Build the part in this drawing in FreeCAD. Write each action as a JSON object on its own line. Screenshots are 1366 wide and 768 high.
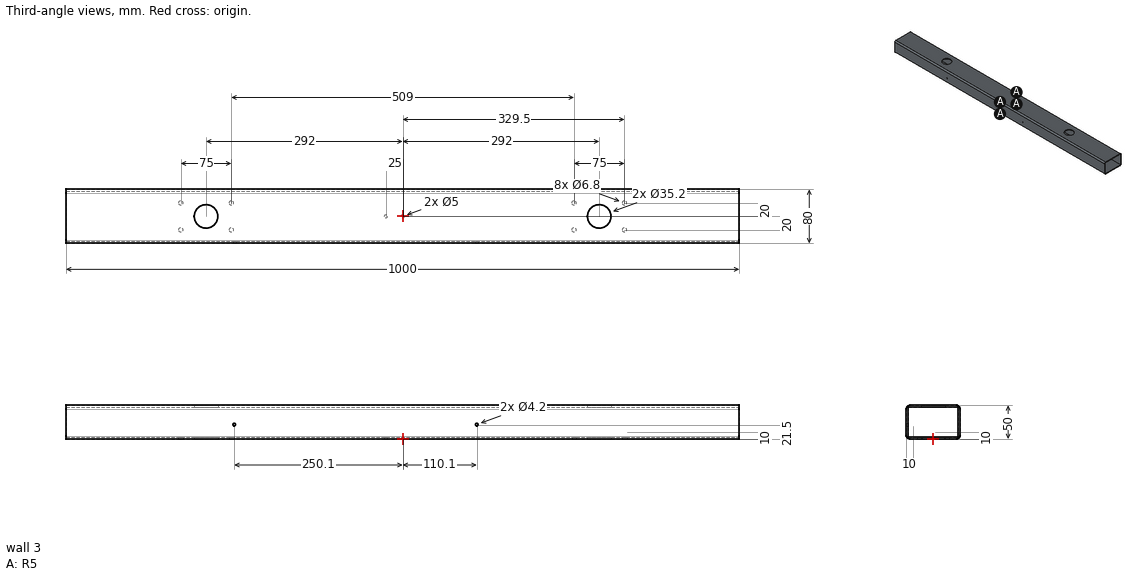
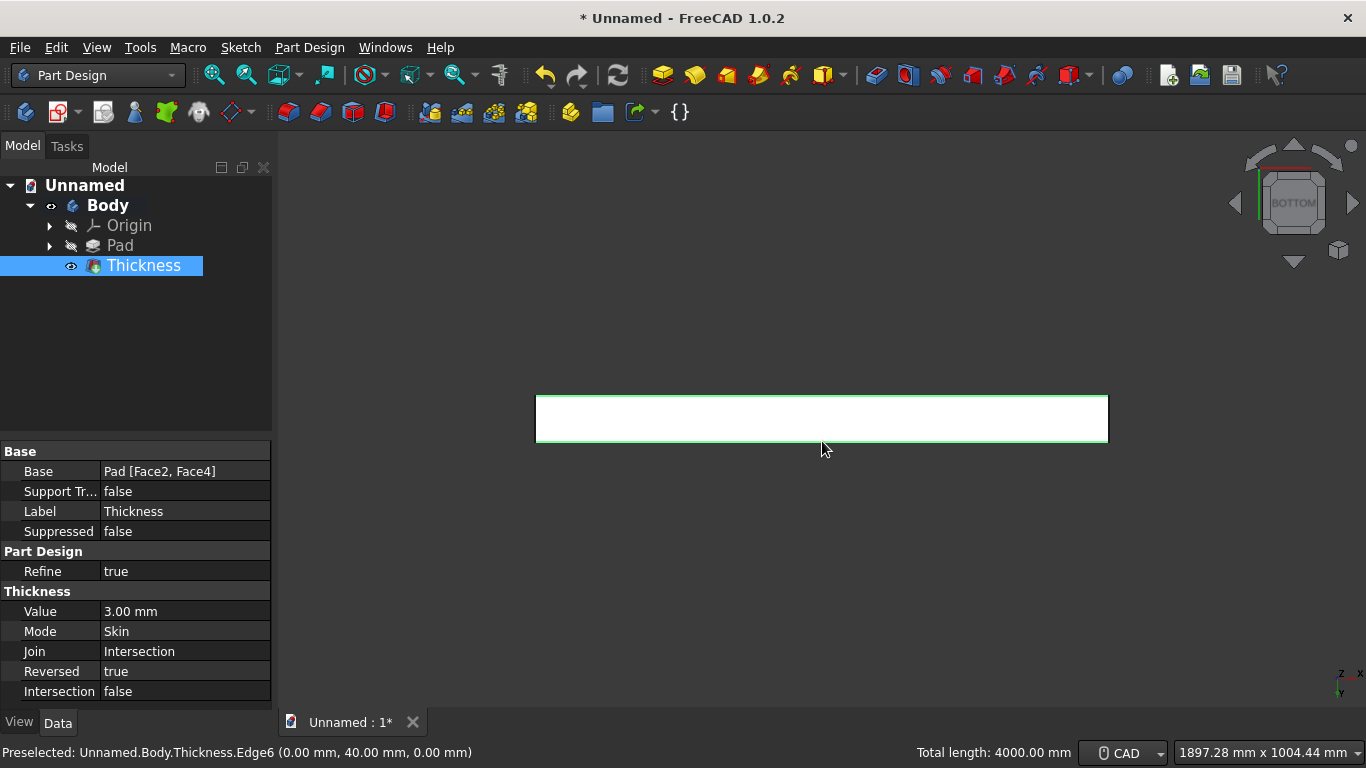
{"action": "left_click", "coordinate": [290, 112]}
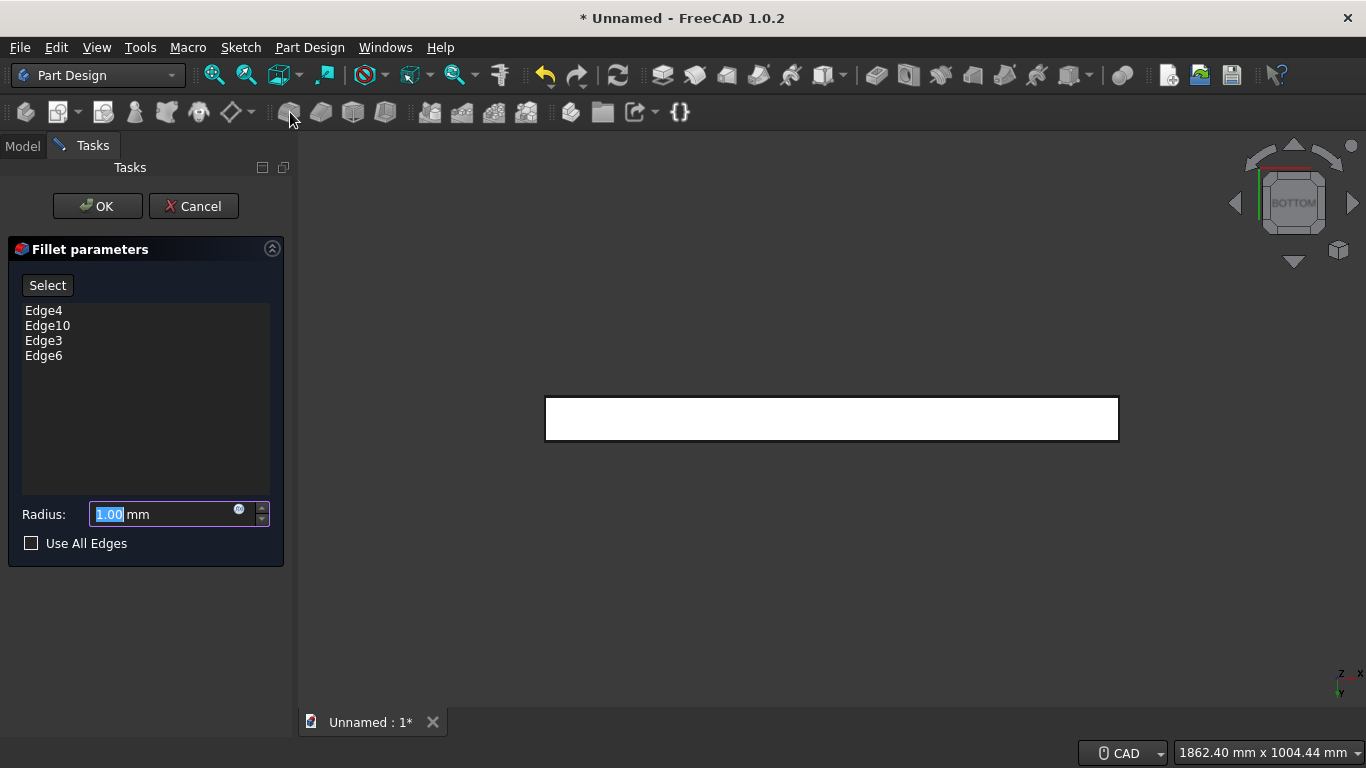
{"action": "type", "text": "5"}
{"action": "key", "text": "Tab"}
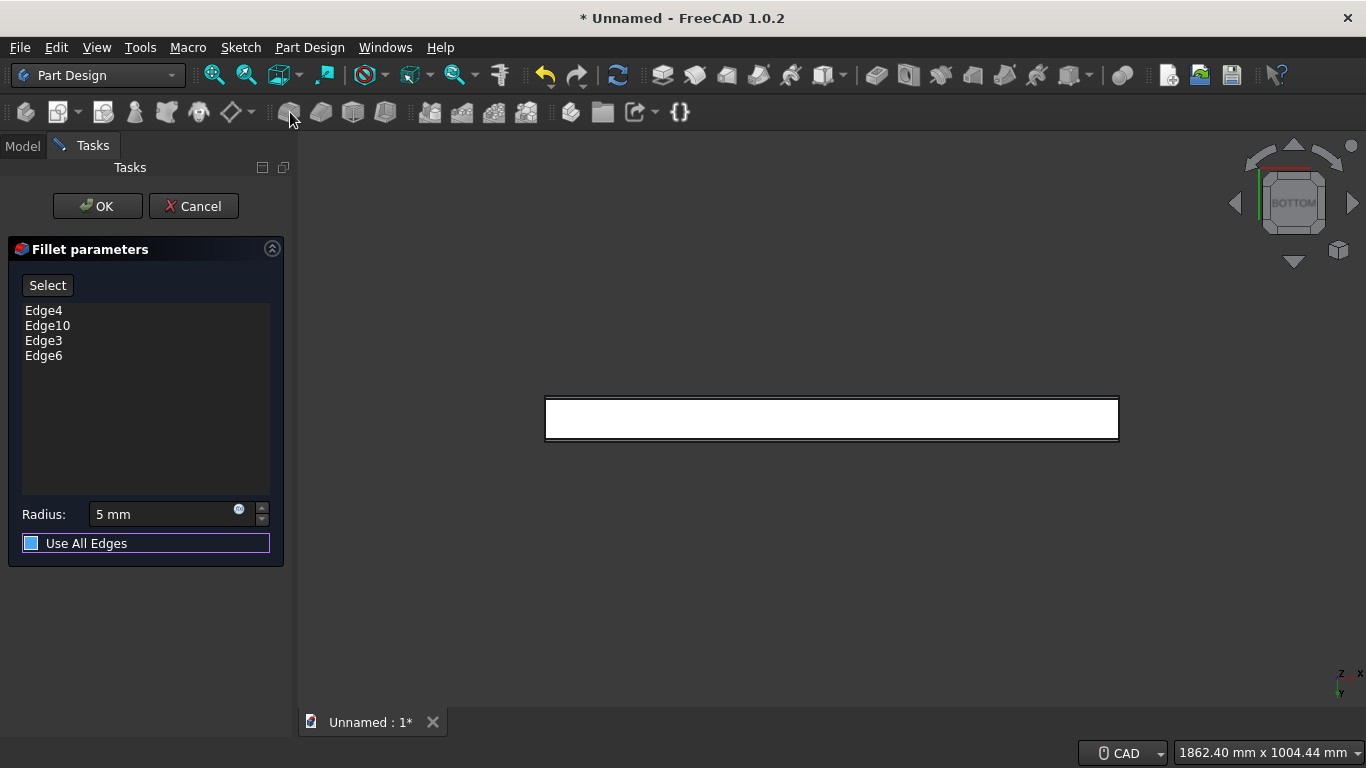
{"action": "left_click", "coordinate": [98, 206]}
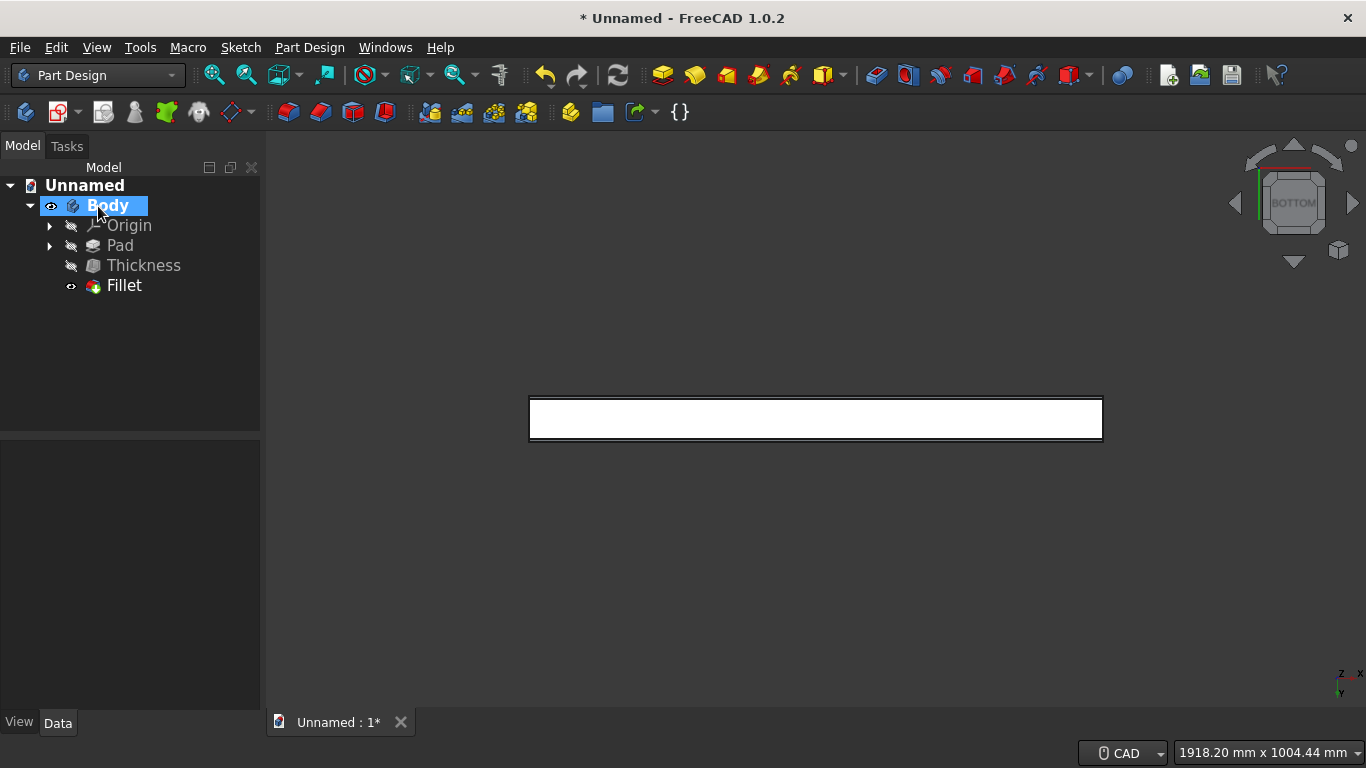
{"action": "left_click", "coordinate": [1062, 418]}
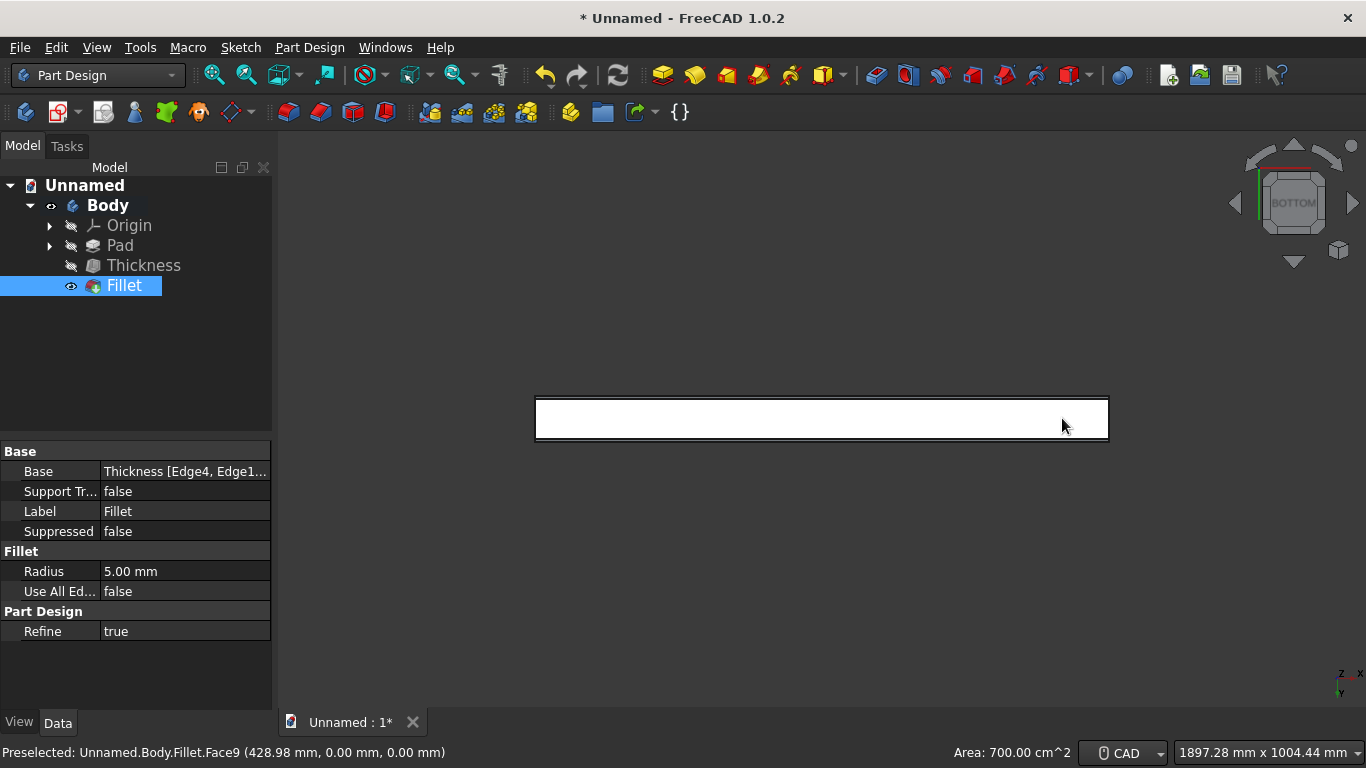
{"action": "left_click", "coordinate": [58, 112]}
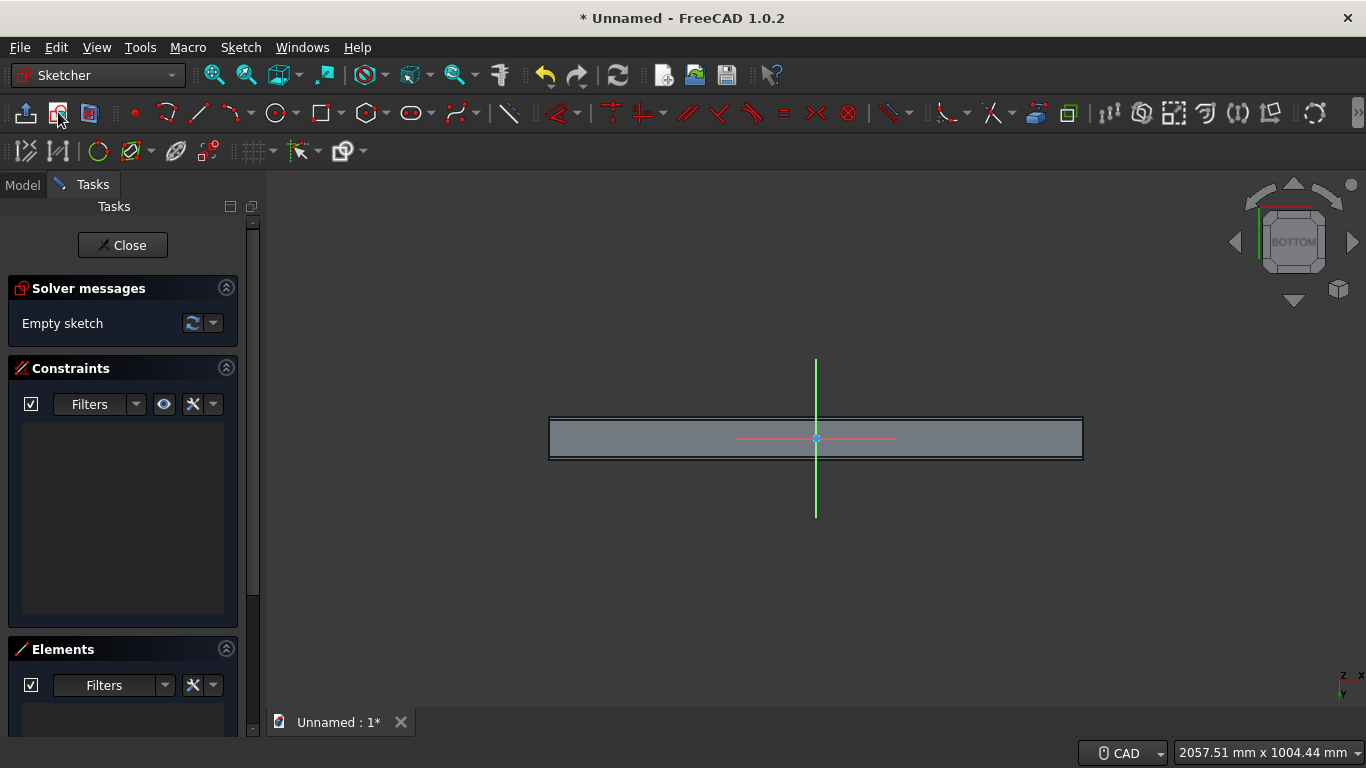
{"action": "scroll", "coordinate": [899, 438], "scroll_direction": "up", "scroll_amount": 3}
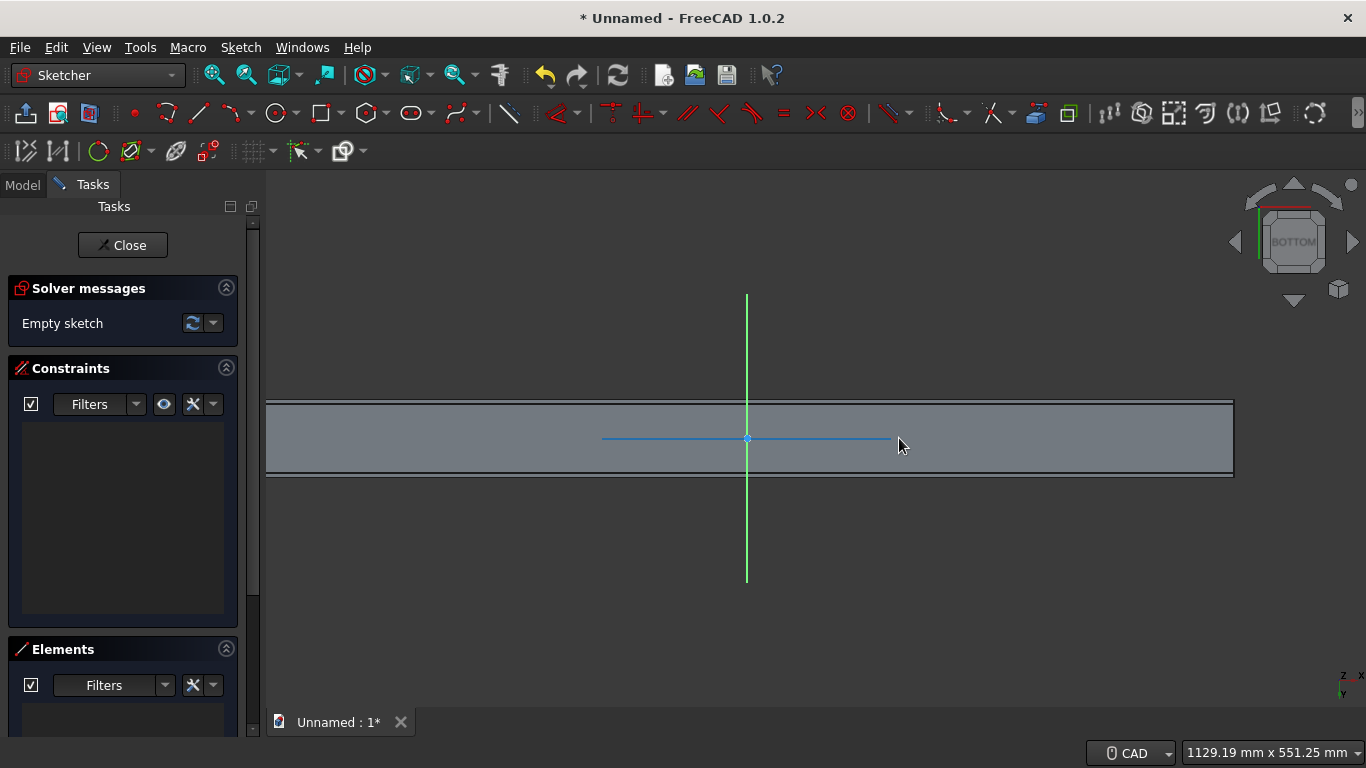
{"action": "key", "text": "g c"}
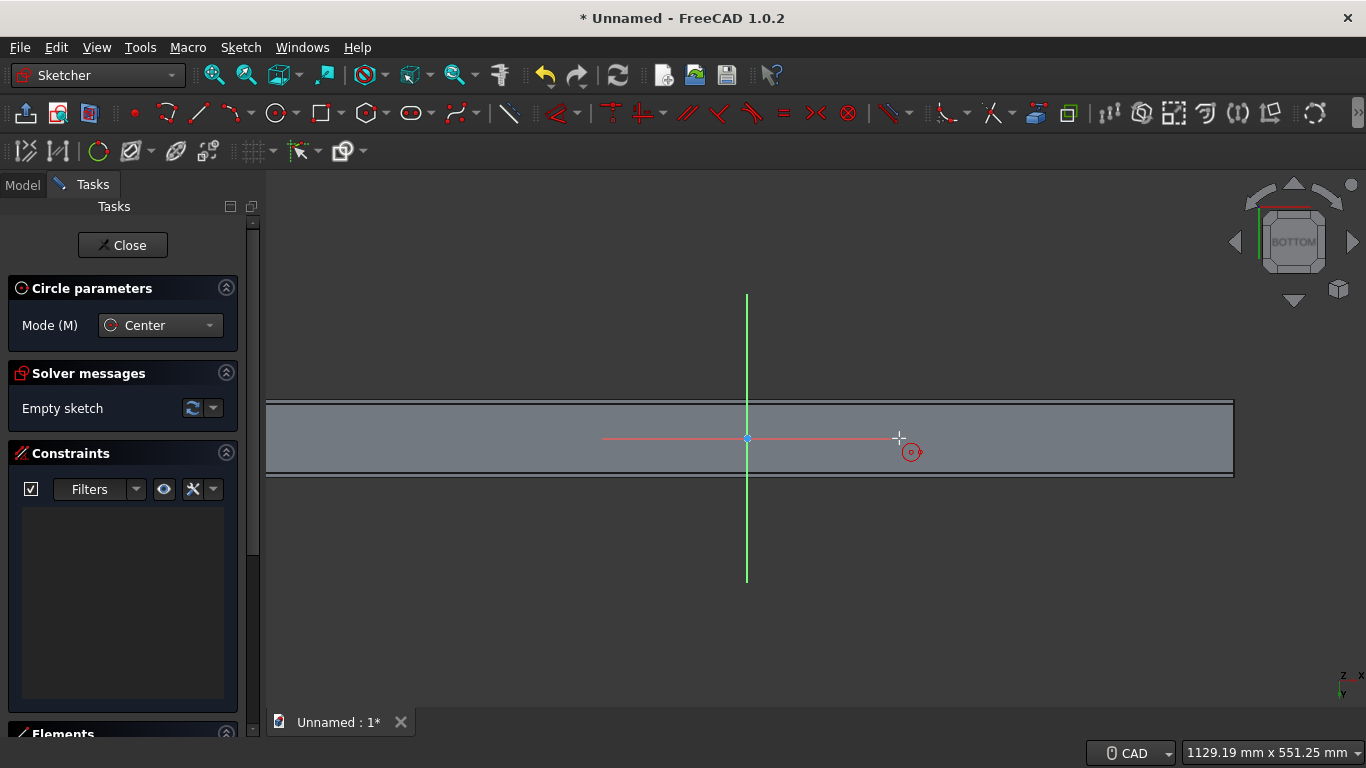
{"action": "scroll", "coordinate": [1032, 438], "scroll_direction": "up", "scroll_amount": 2}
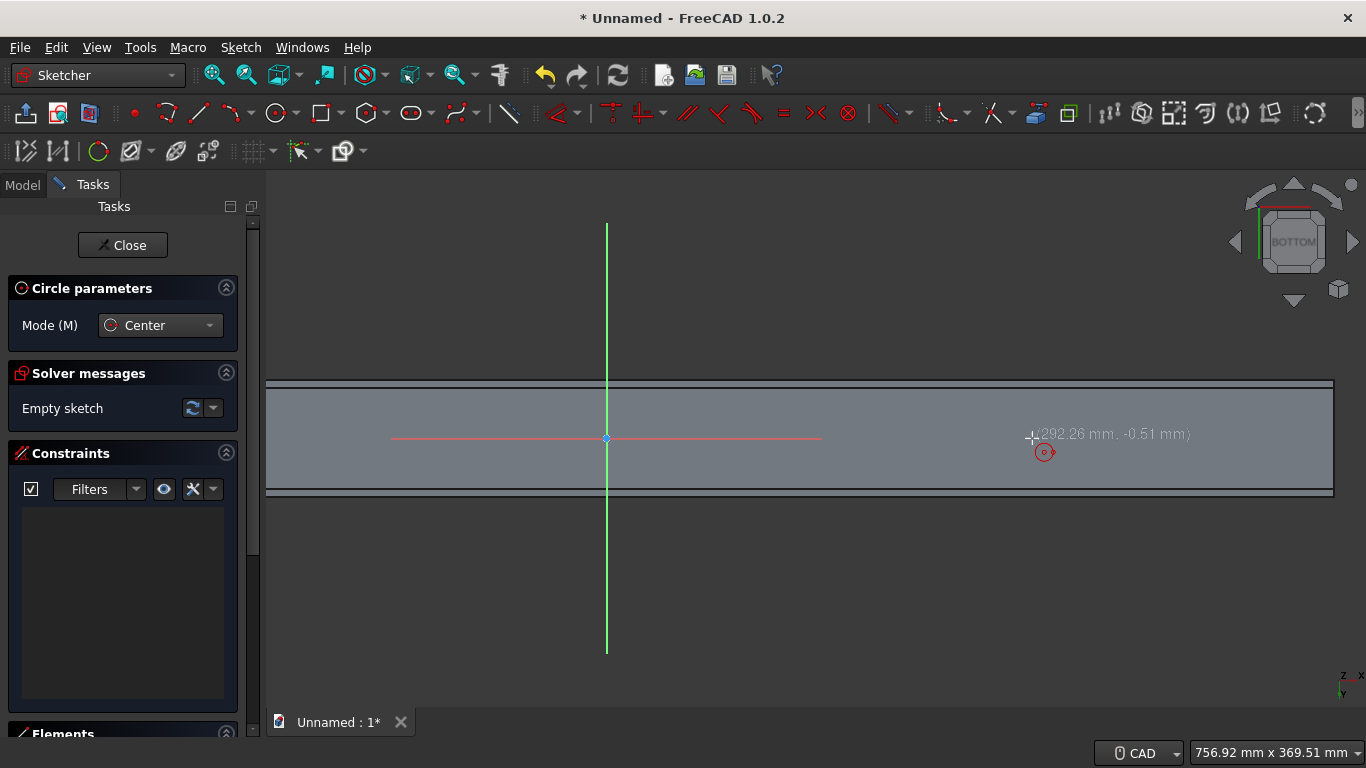
{"action": "left_click", "coordinate": [1031, 438]}
{"action": "mouse_move", "coordinate": [1049, 420]}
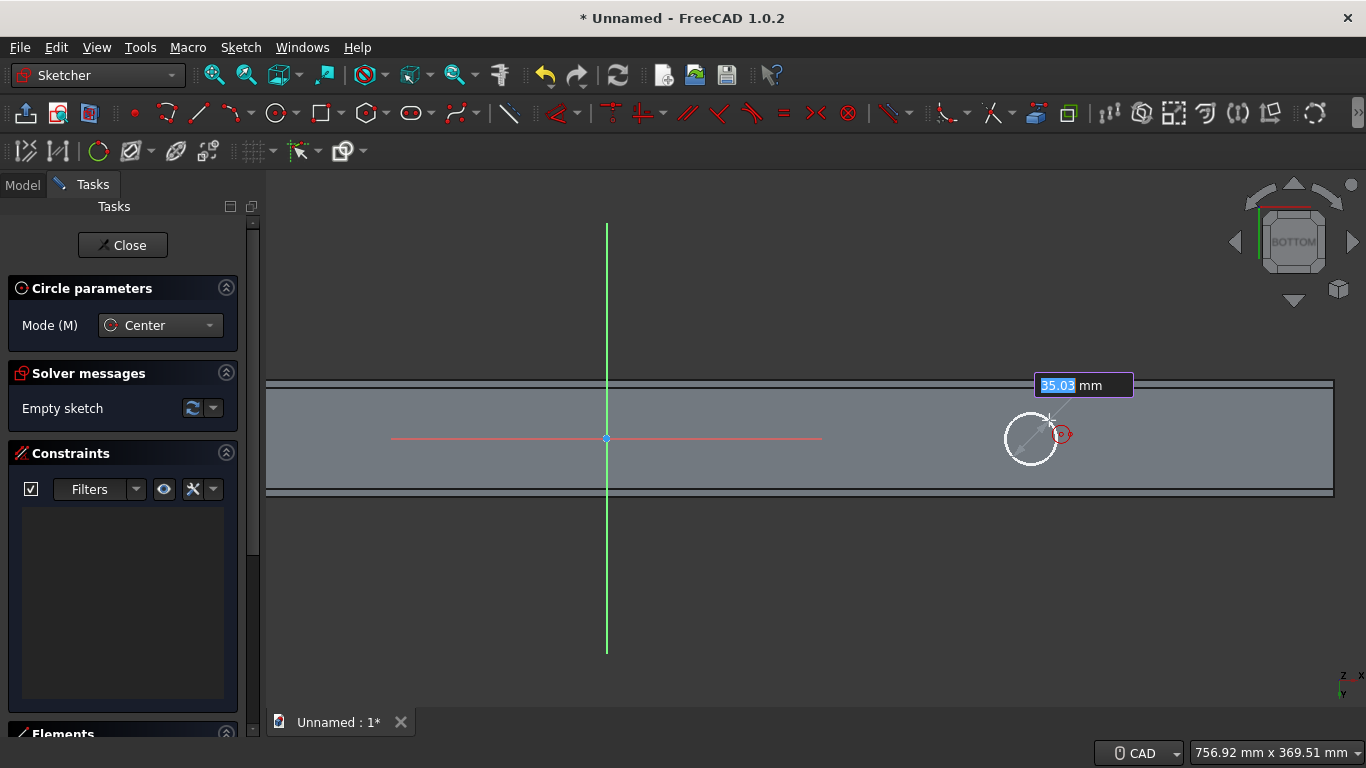
{"action": "type", "text": "35.2"}
{"action": "key", "text": "Return"}